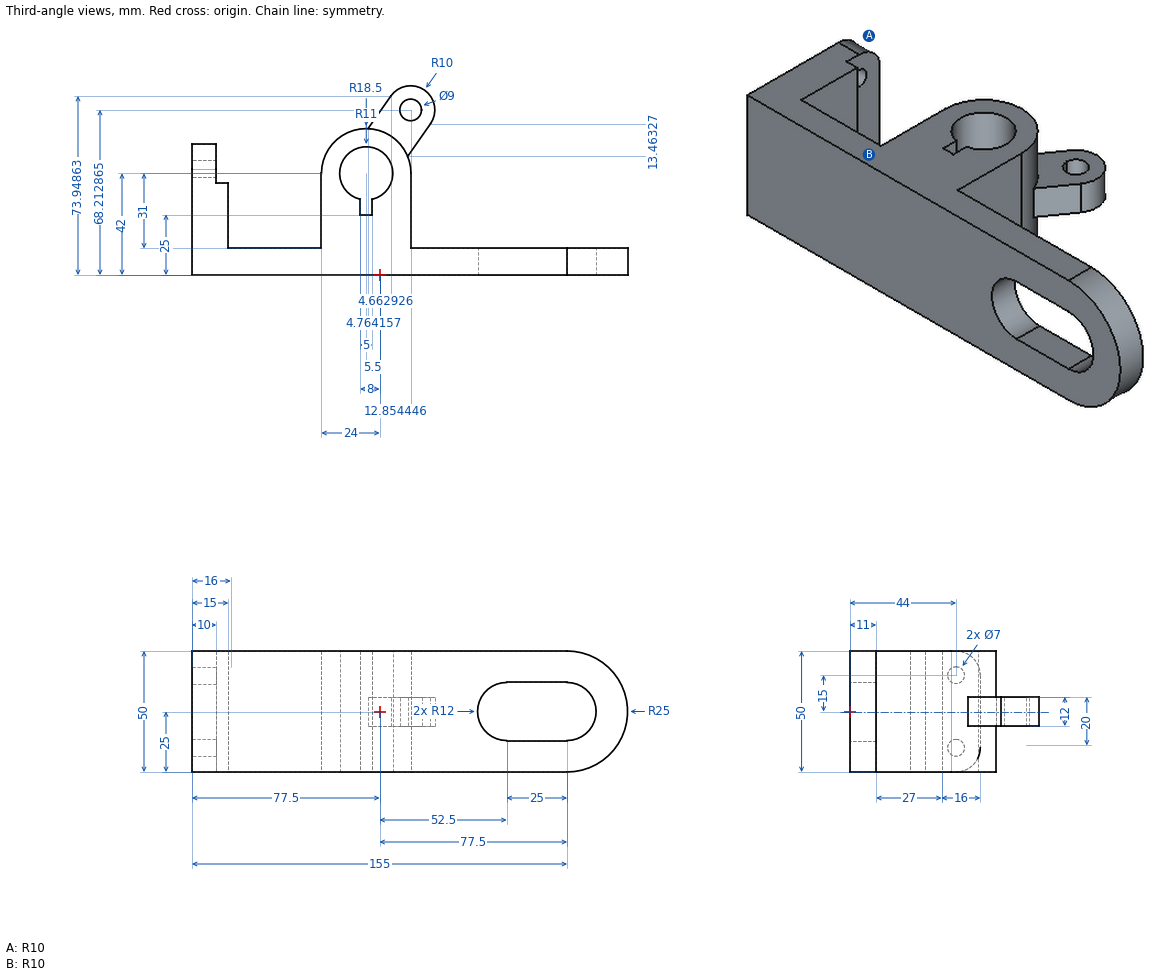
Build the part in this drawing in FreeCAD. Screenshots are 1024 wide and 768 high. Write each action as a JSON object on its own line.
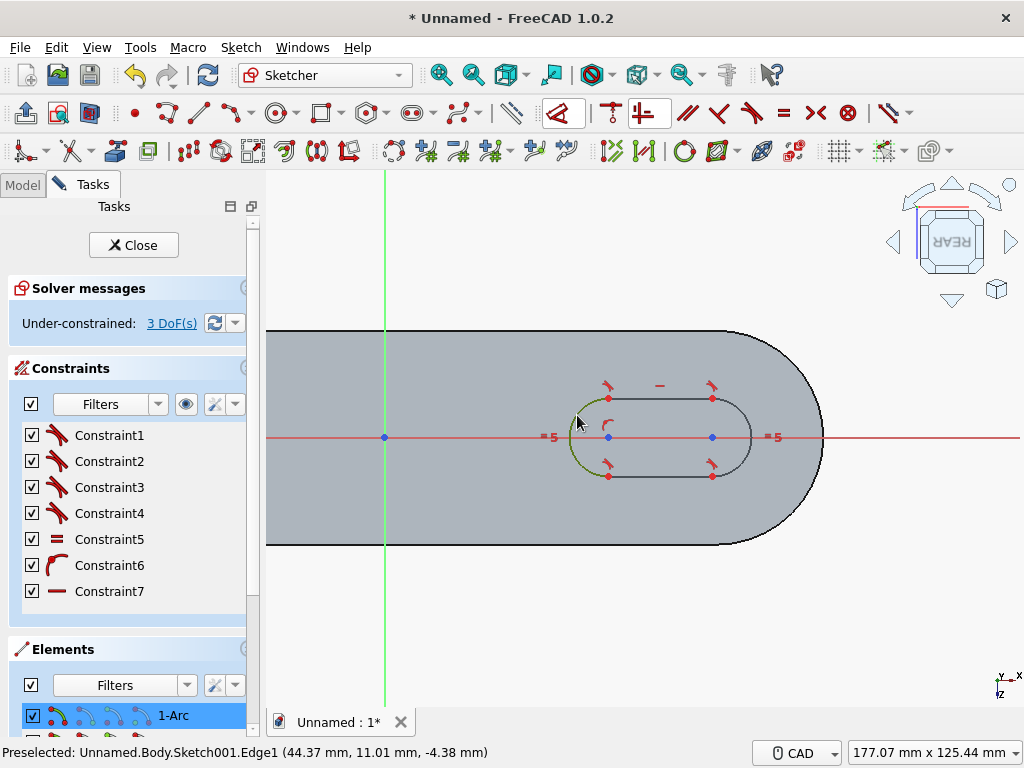
{"action": "key", "text": "k r"}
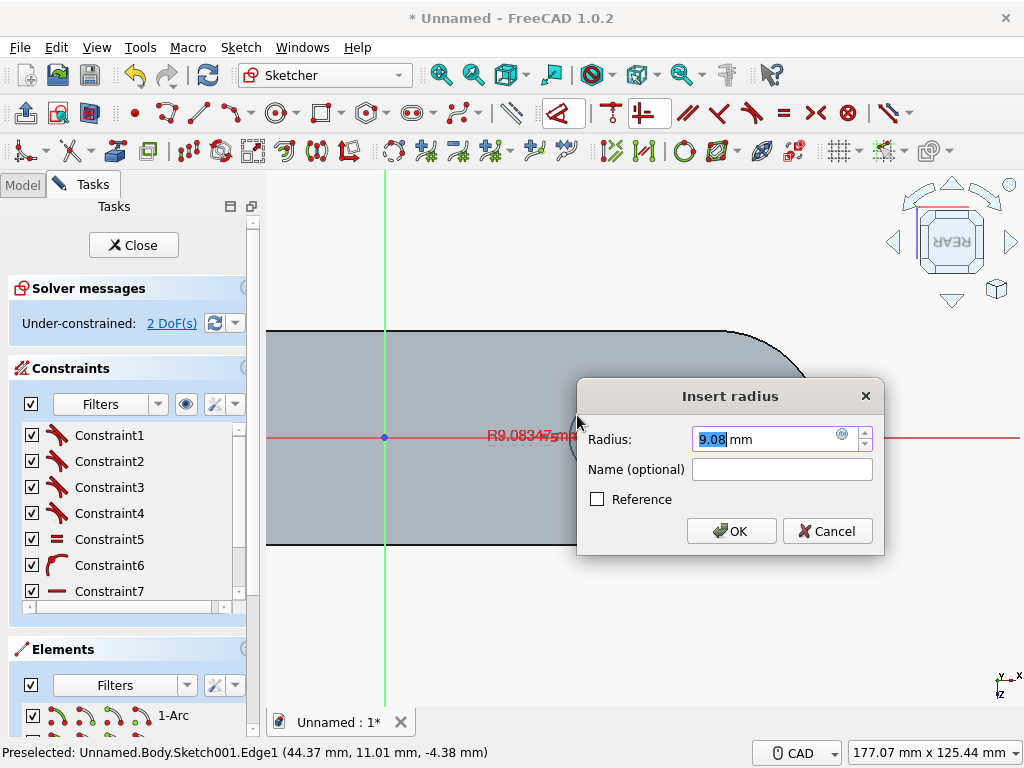
{"action": "type", "text": "12"}
{"action": "key", "text": "Return"}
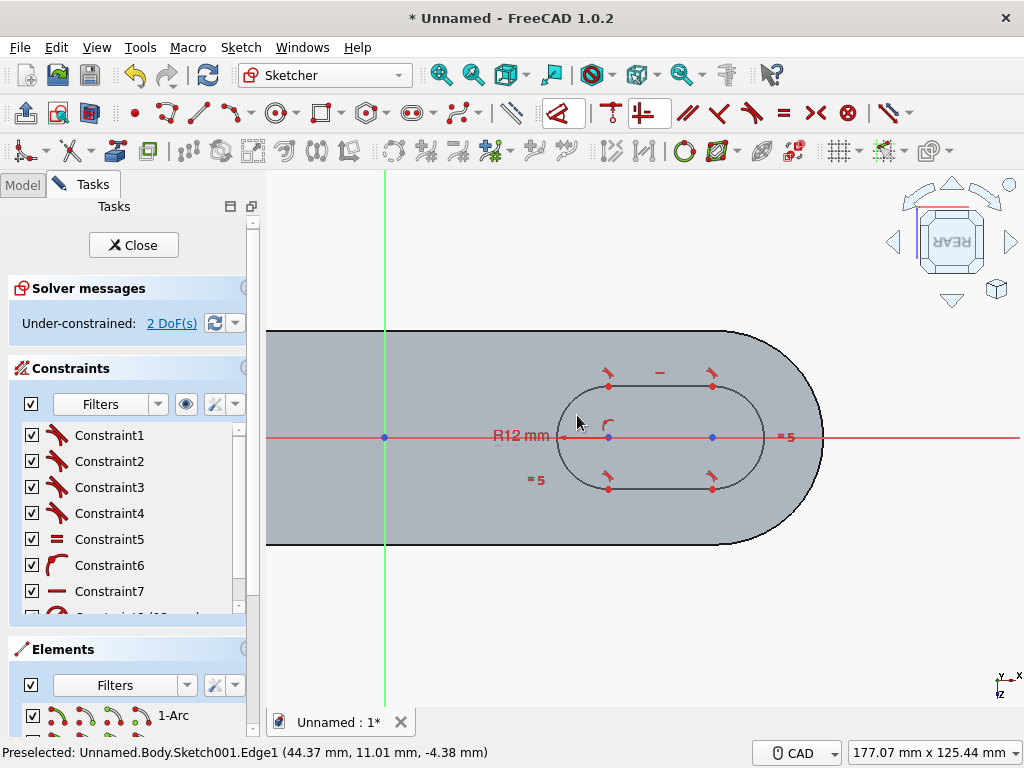
{"action": "left_click", "coordinate": [640, 386]}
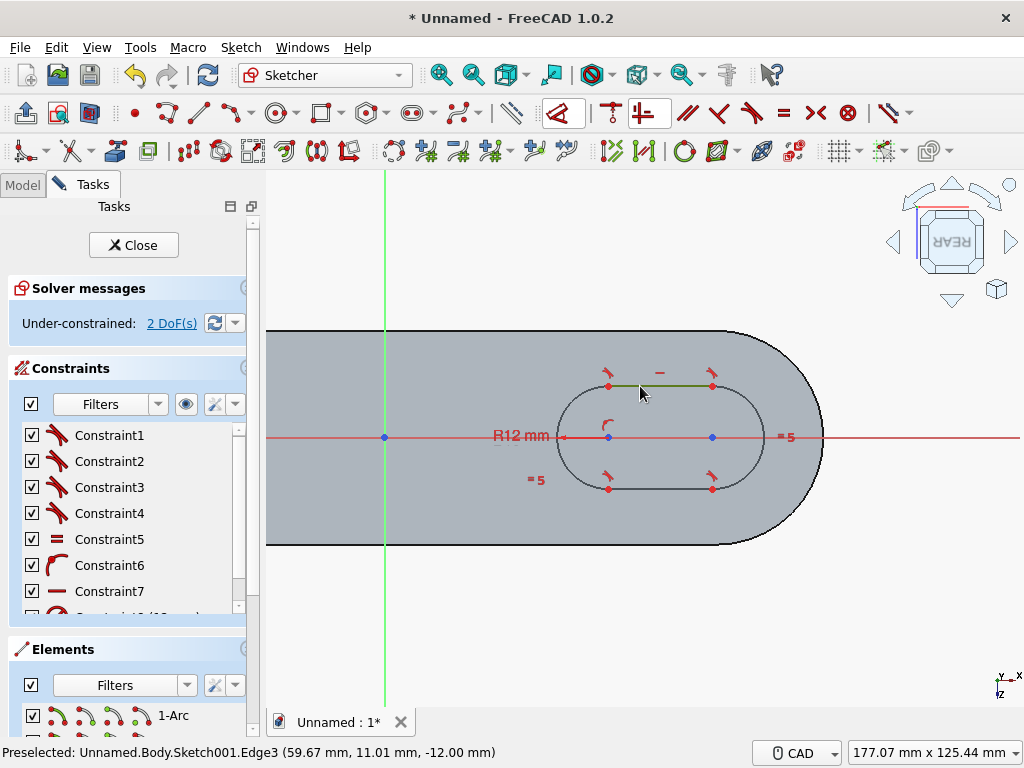
{"action": "key", "text": "l"}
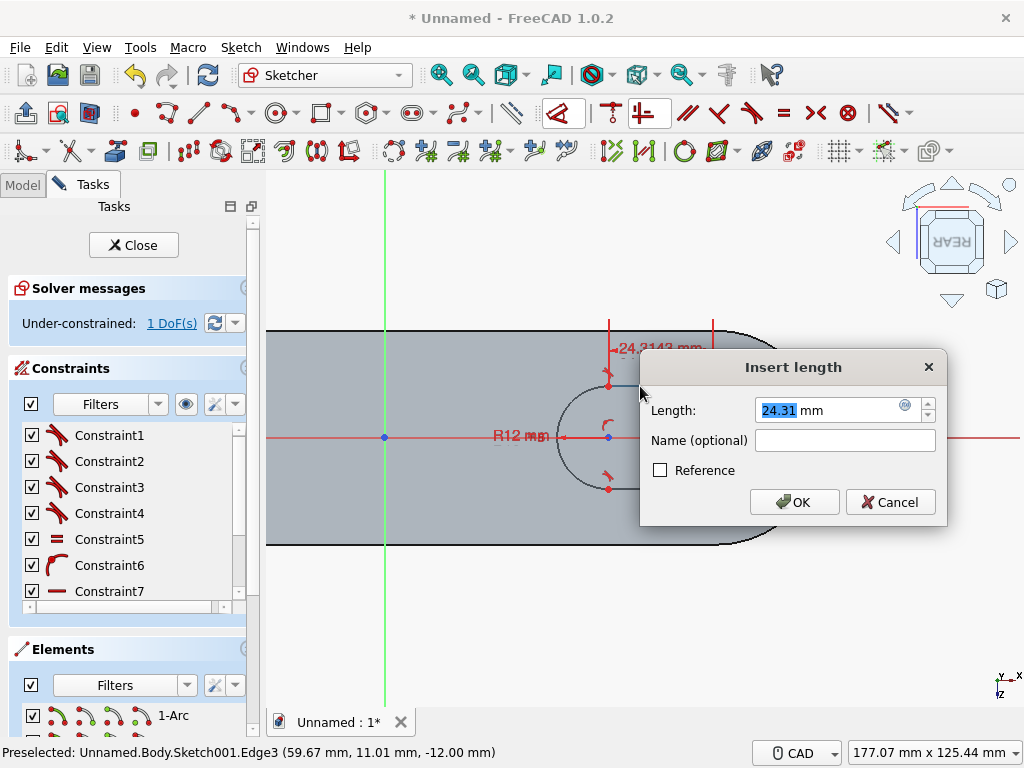
{"action": "type", "text": "25"}
{"action": "key", "text": "Return"}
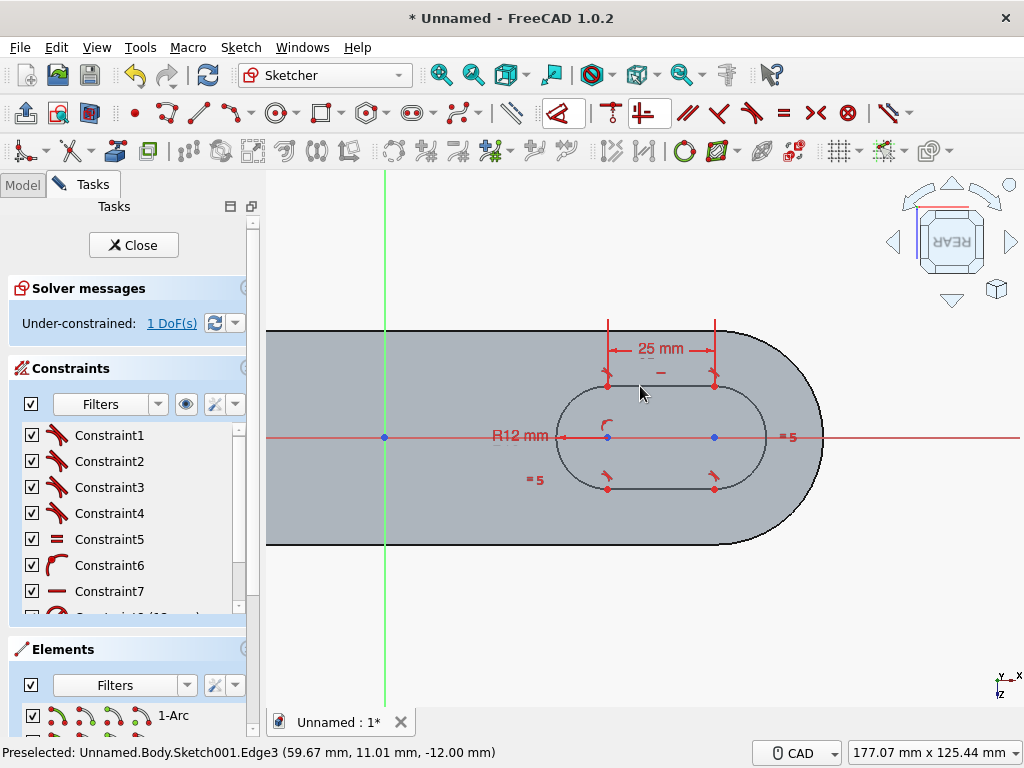
{"action": "left_click", "coordinate": [608, 386]}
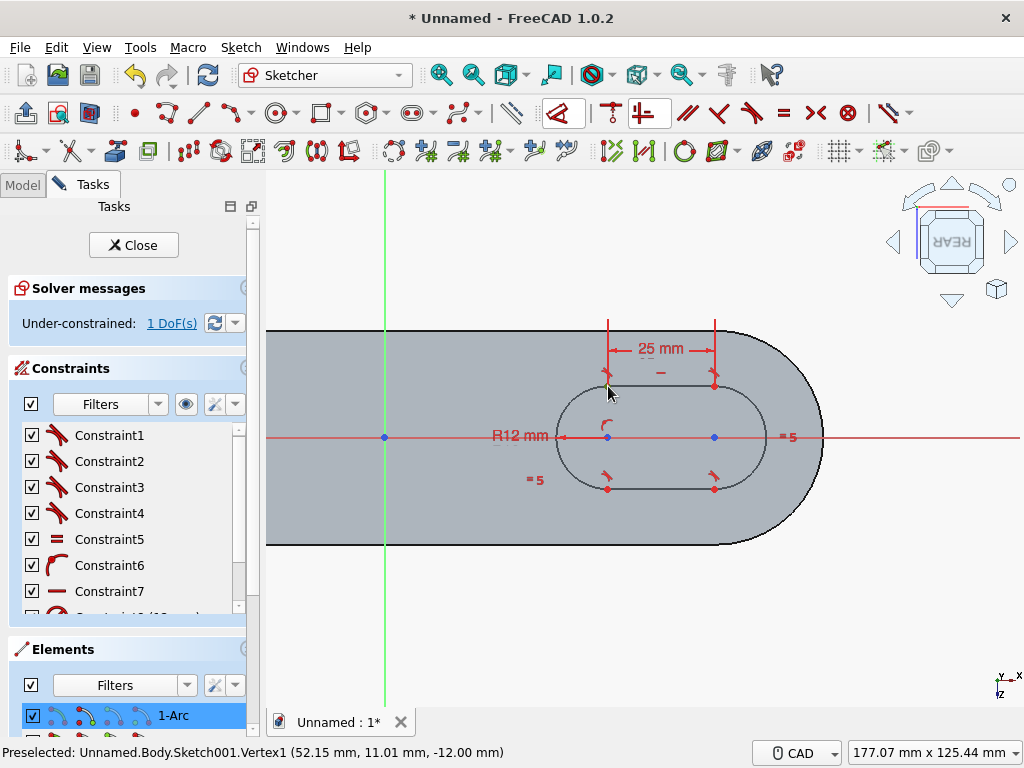
{"action": "left_click", "coordinate": [580, 114]}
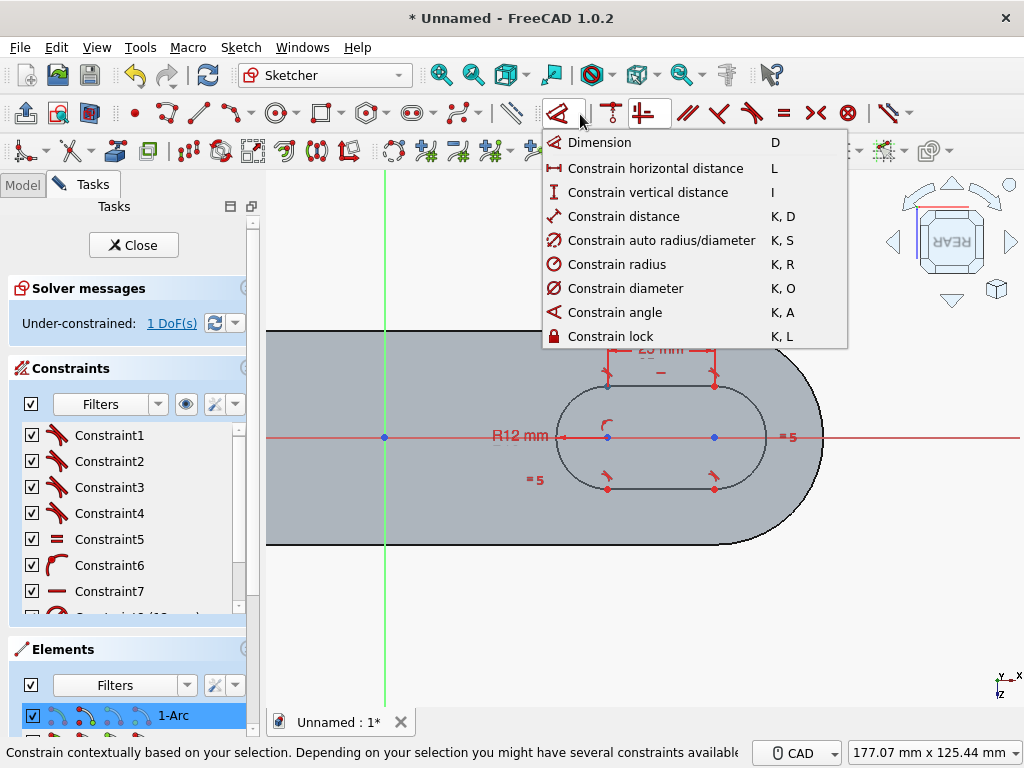
{"action": "left_click", "coordinate": [695, 168]}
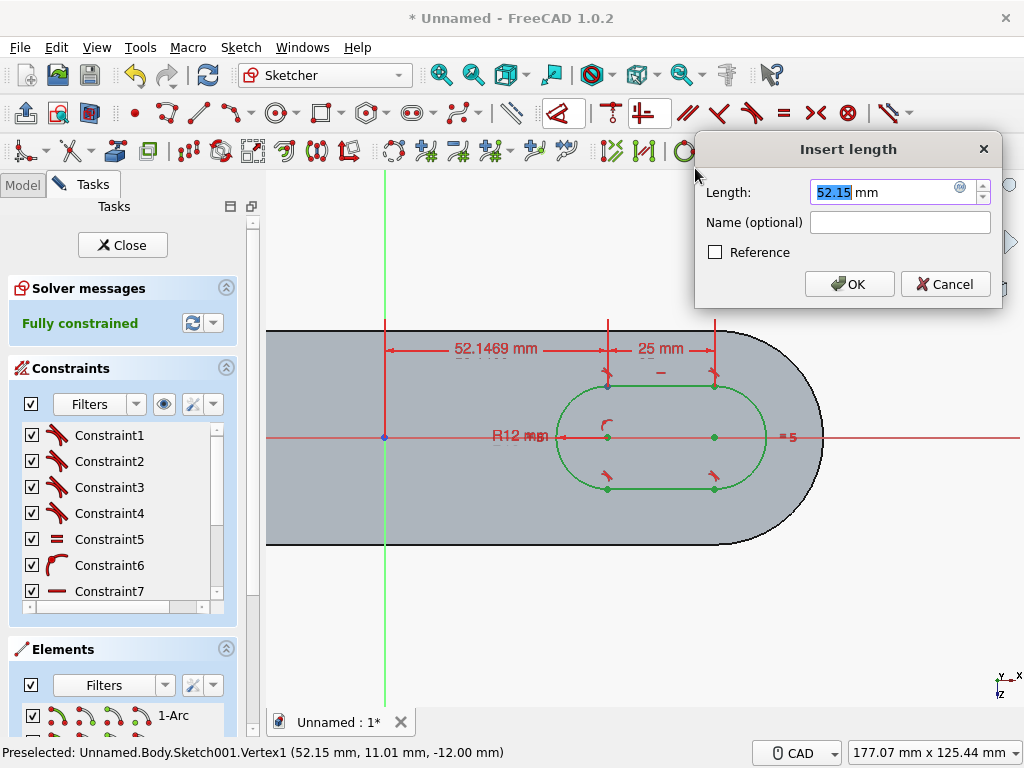
{"action": "type", "text": "52.5"}
{"action": "key", "text": "Return"}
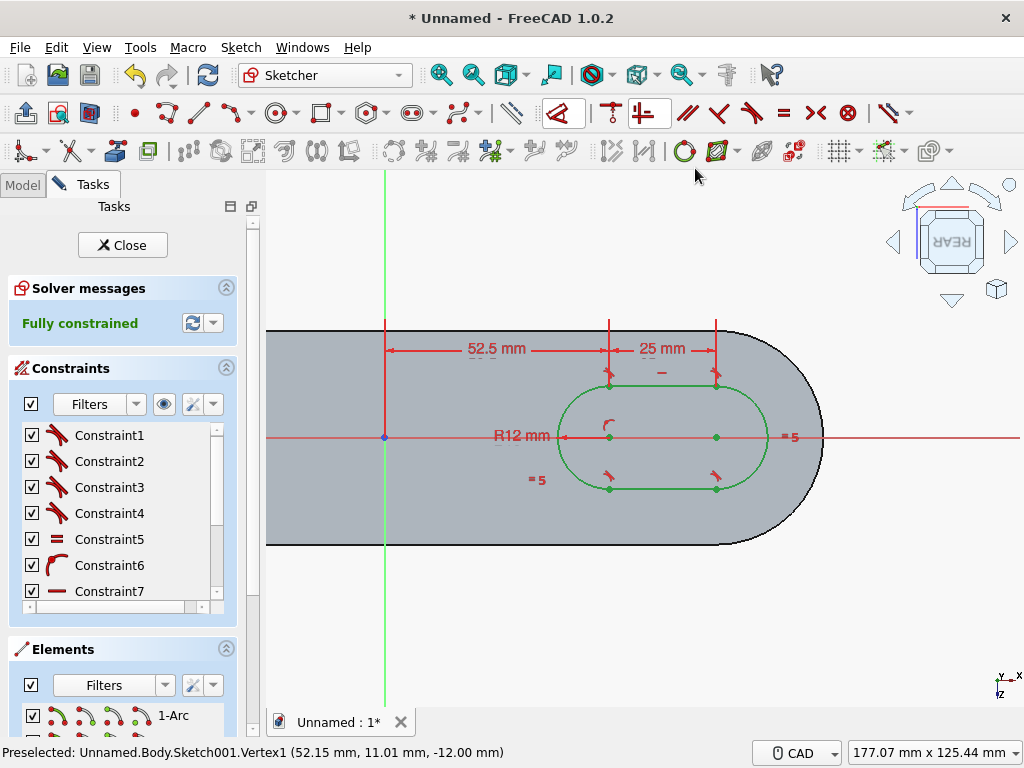
{"action": "left_click", "coordinate": [123, 245]}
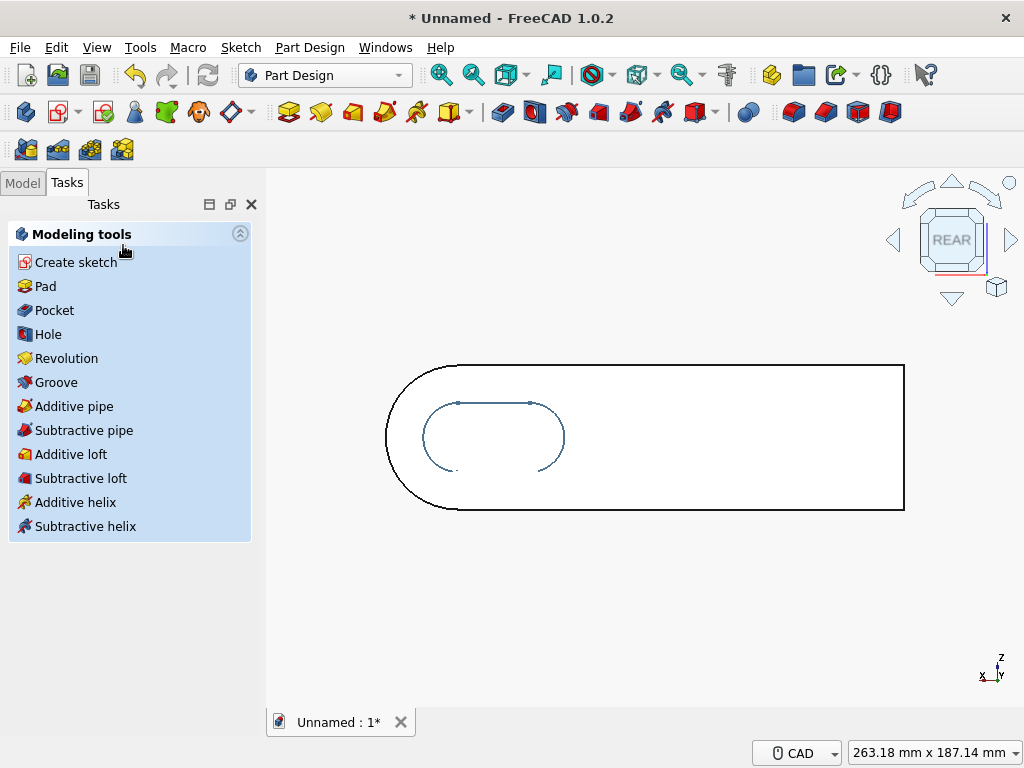
{"action": "left_click", "coordinate": [504, 112]}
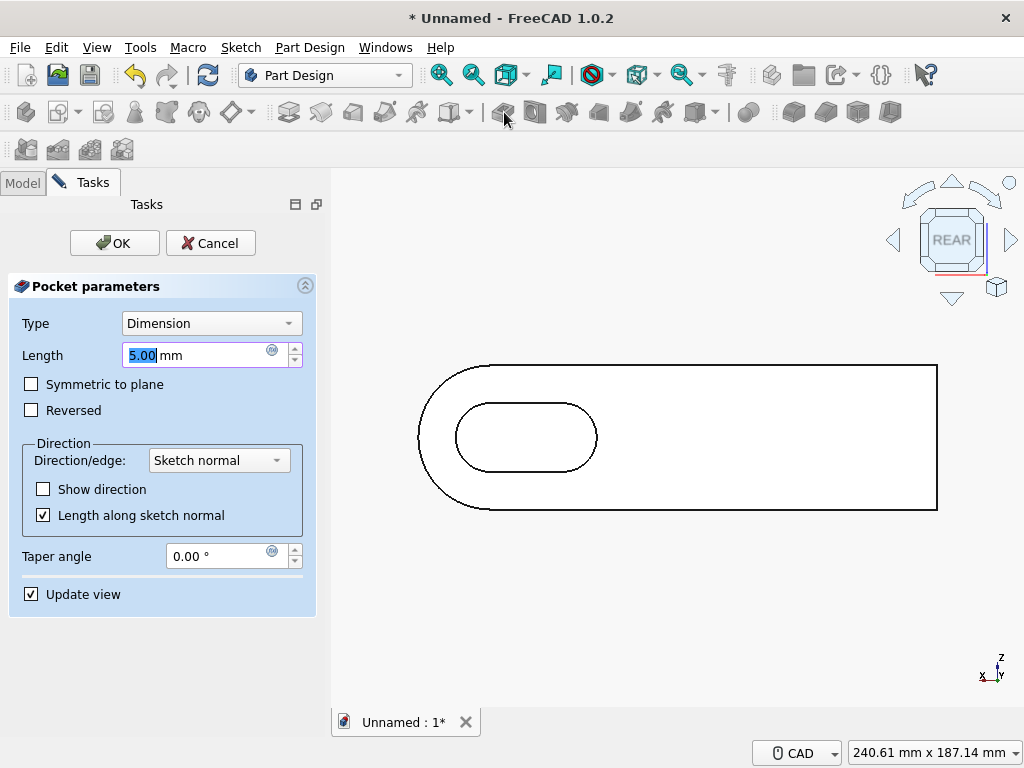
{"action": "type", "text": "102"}
{"action": "key", "text": "Tab"}